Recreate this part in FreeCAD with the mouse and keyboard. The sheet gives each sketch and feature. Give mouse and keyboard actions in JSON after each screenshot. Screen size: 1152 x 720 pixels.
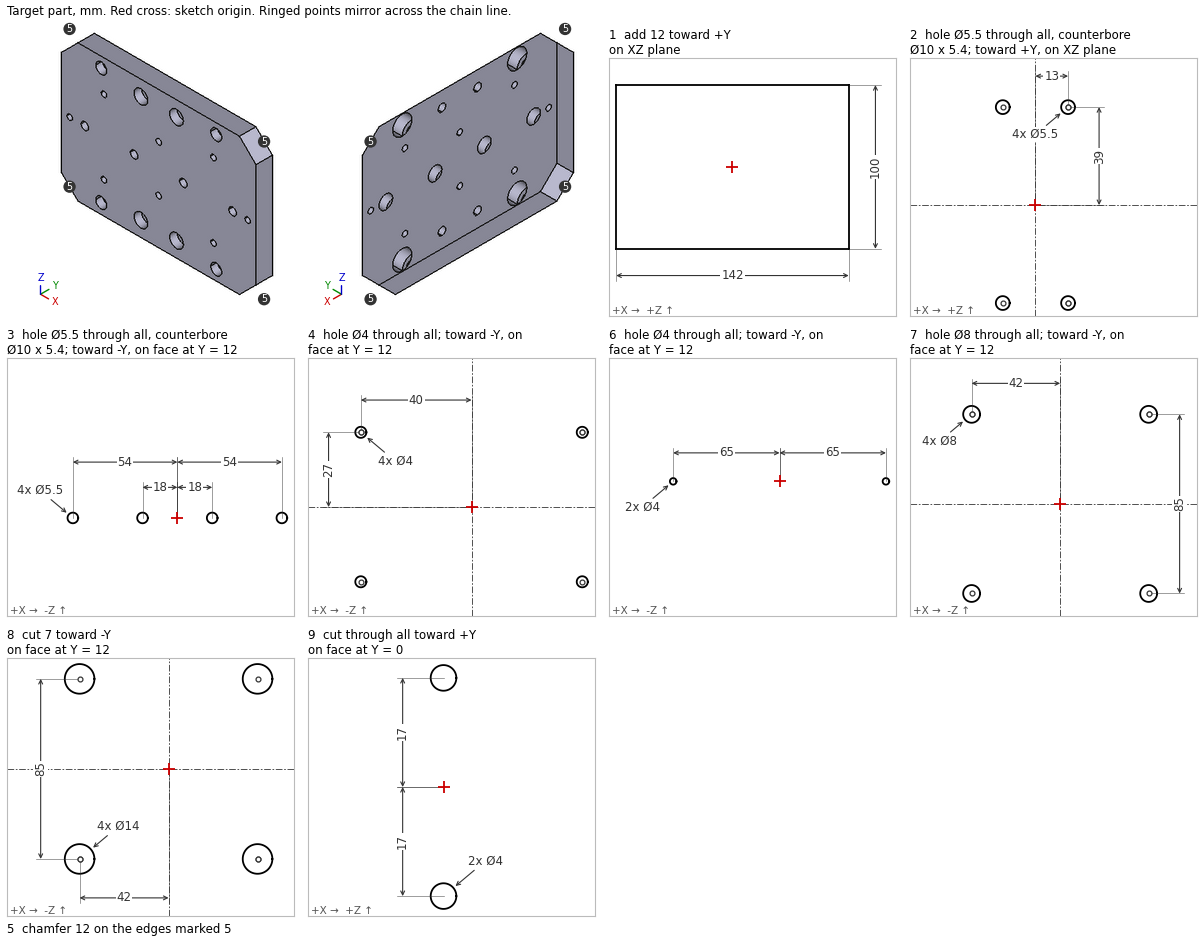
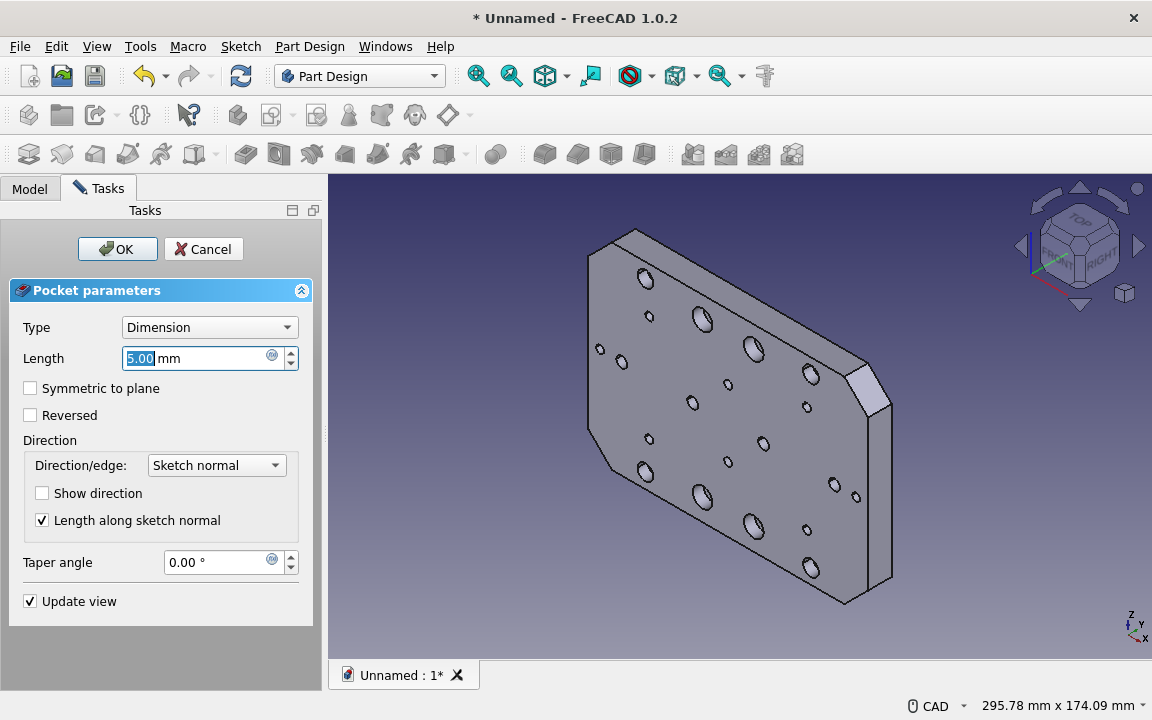
{"action": "left_click", "coordinate": [210, 328]}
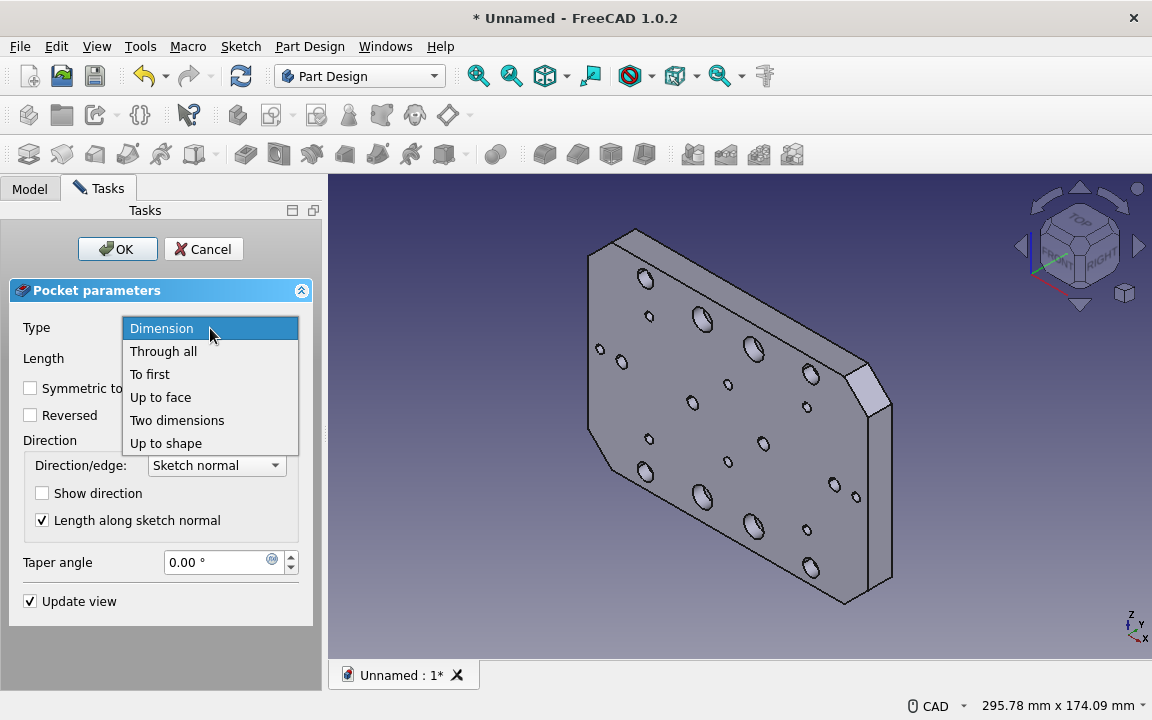
{"action": "left_click", "coordinate": [208, 352]}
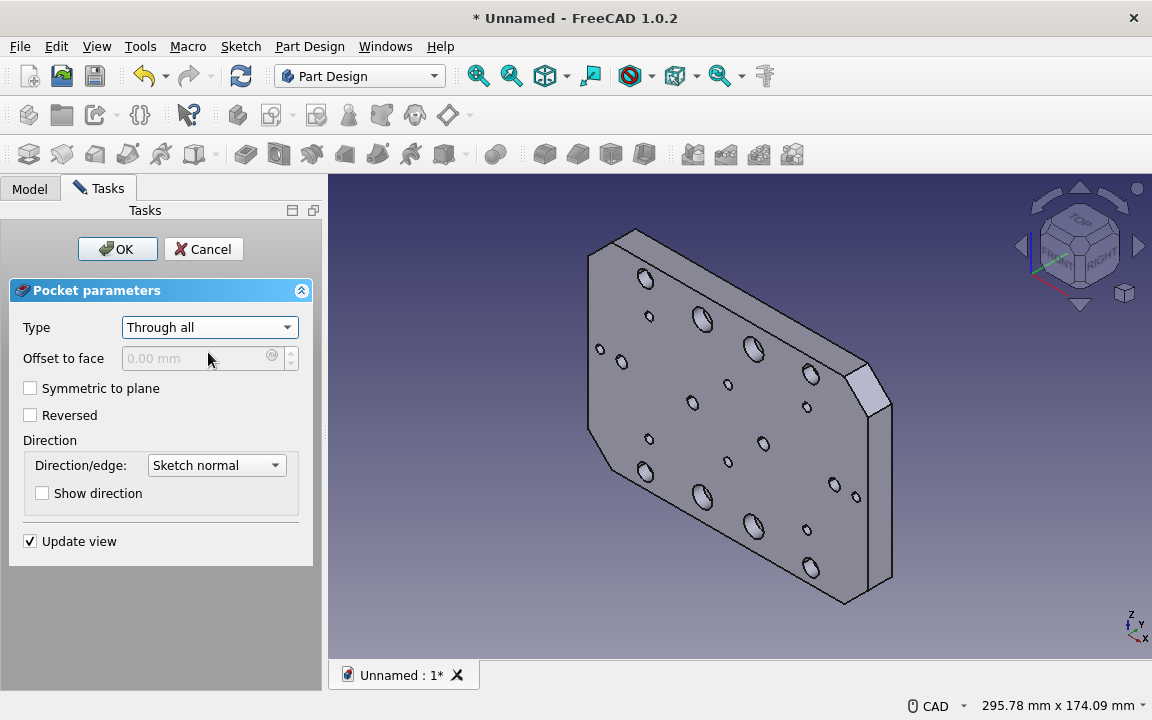
{"action": "left_click", "coordinate": [118, 249]}